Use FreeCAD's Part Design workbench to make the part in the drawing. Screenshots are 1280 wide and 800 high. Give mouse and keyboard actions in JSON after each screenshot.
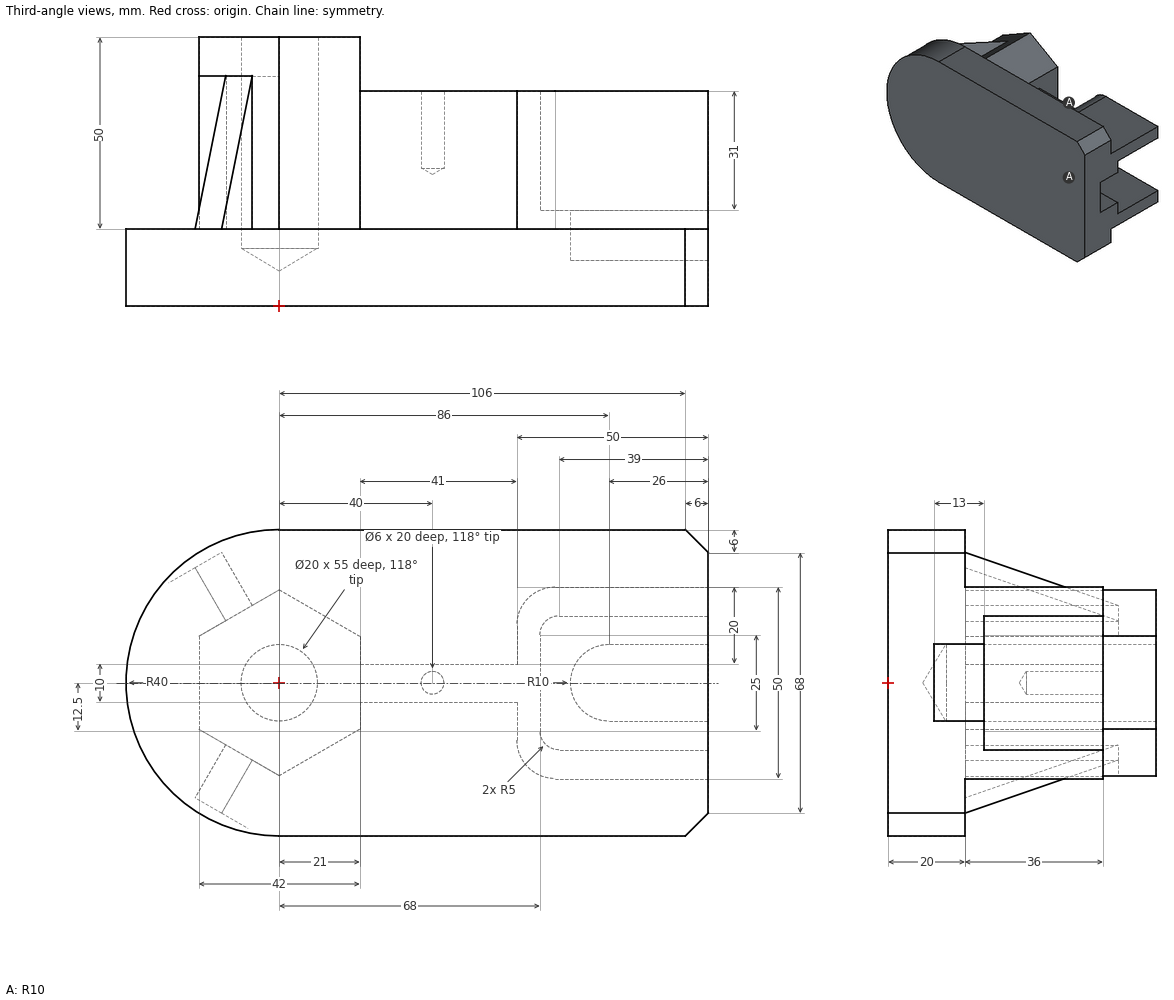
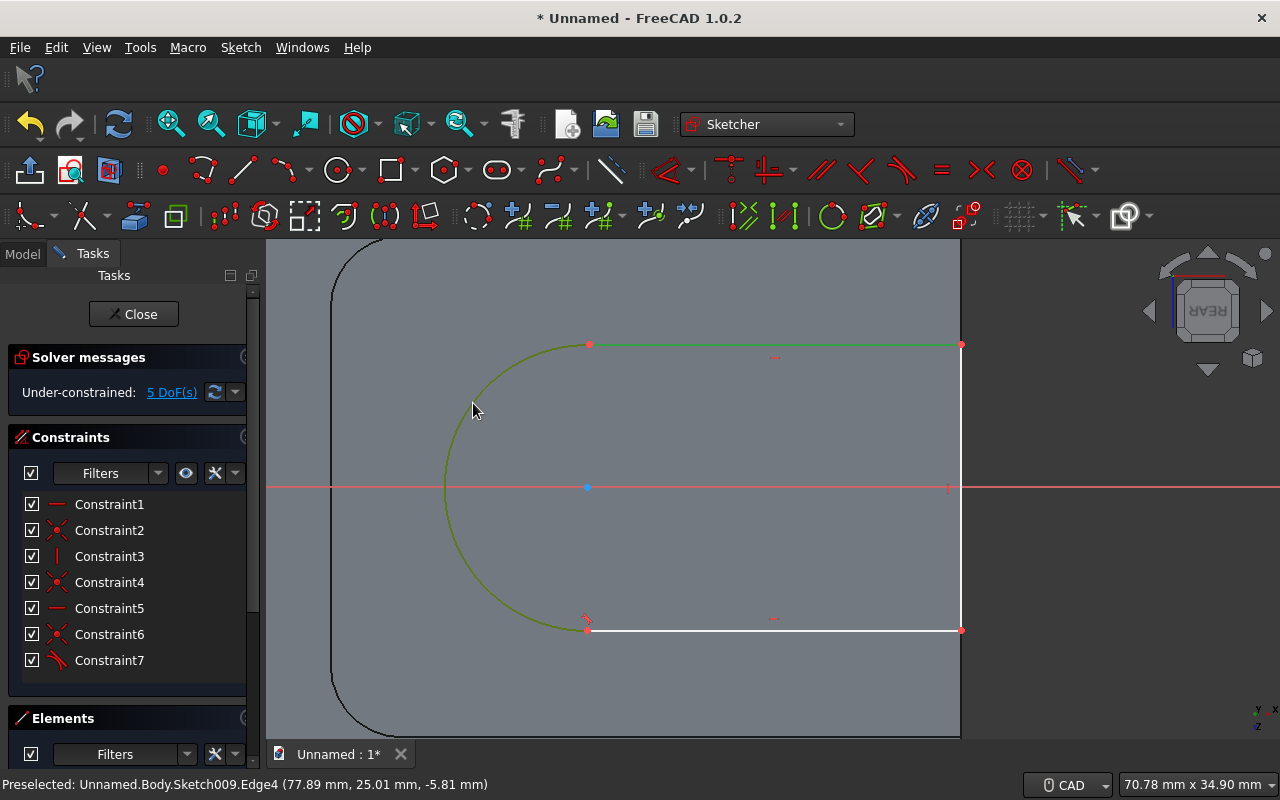
{"action": "left_click", "coordinate": [902, 170]}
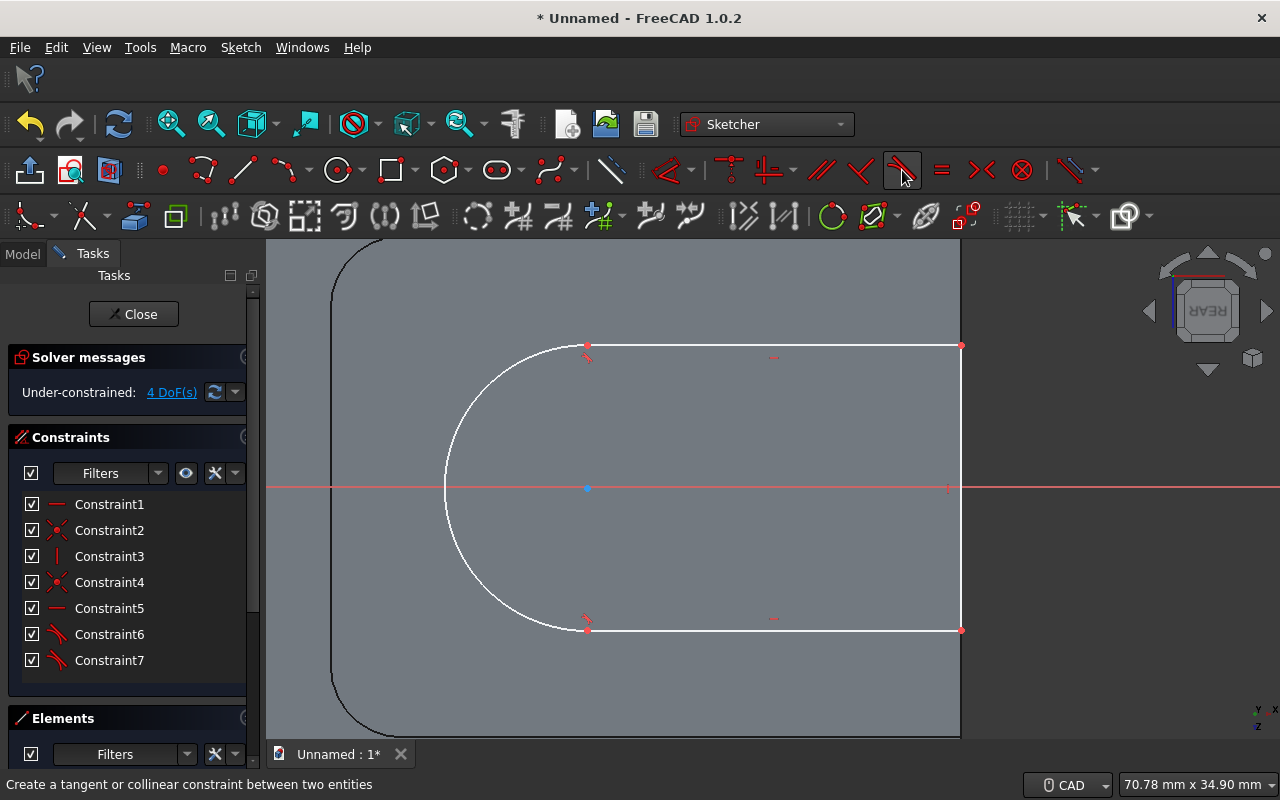
{"action": "left_click", "coordinate": [588, 488]}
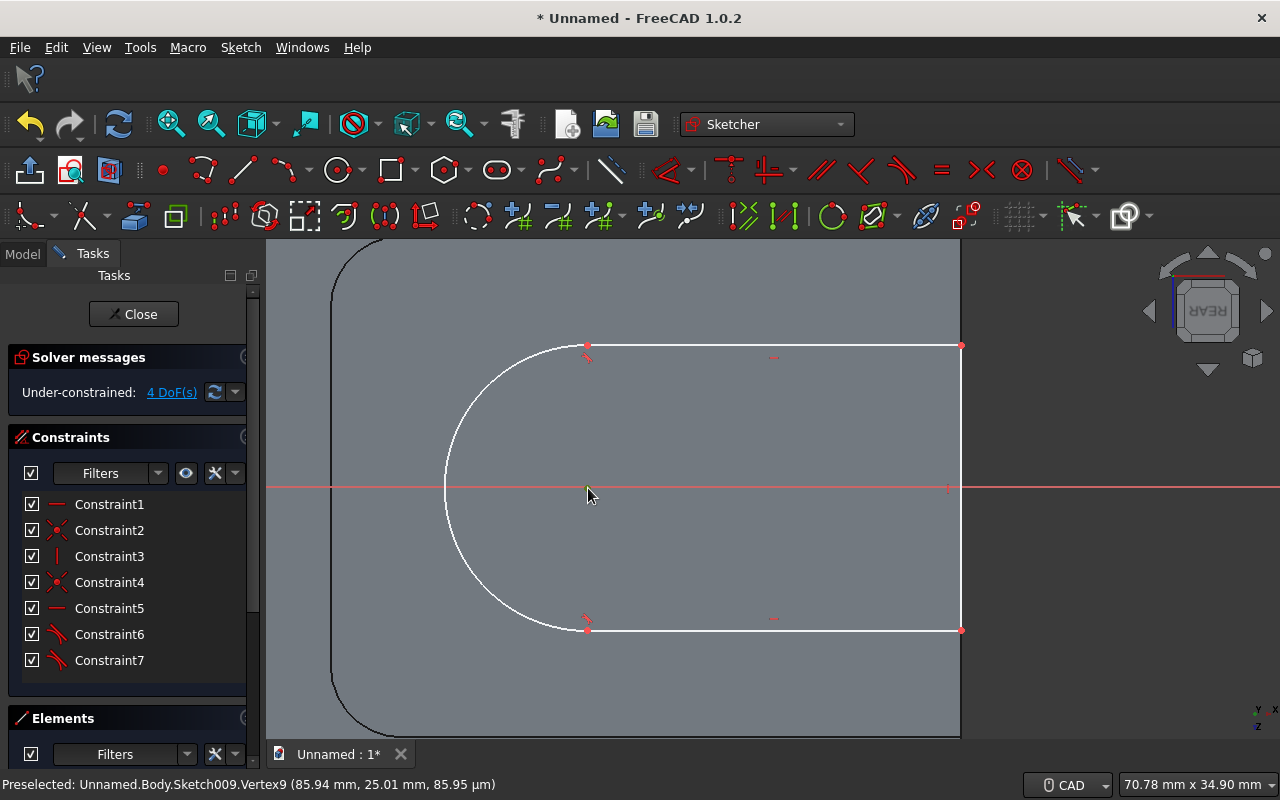
{"action": "left_click", "coordinate": [353, 487]}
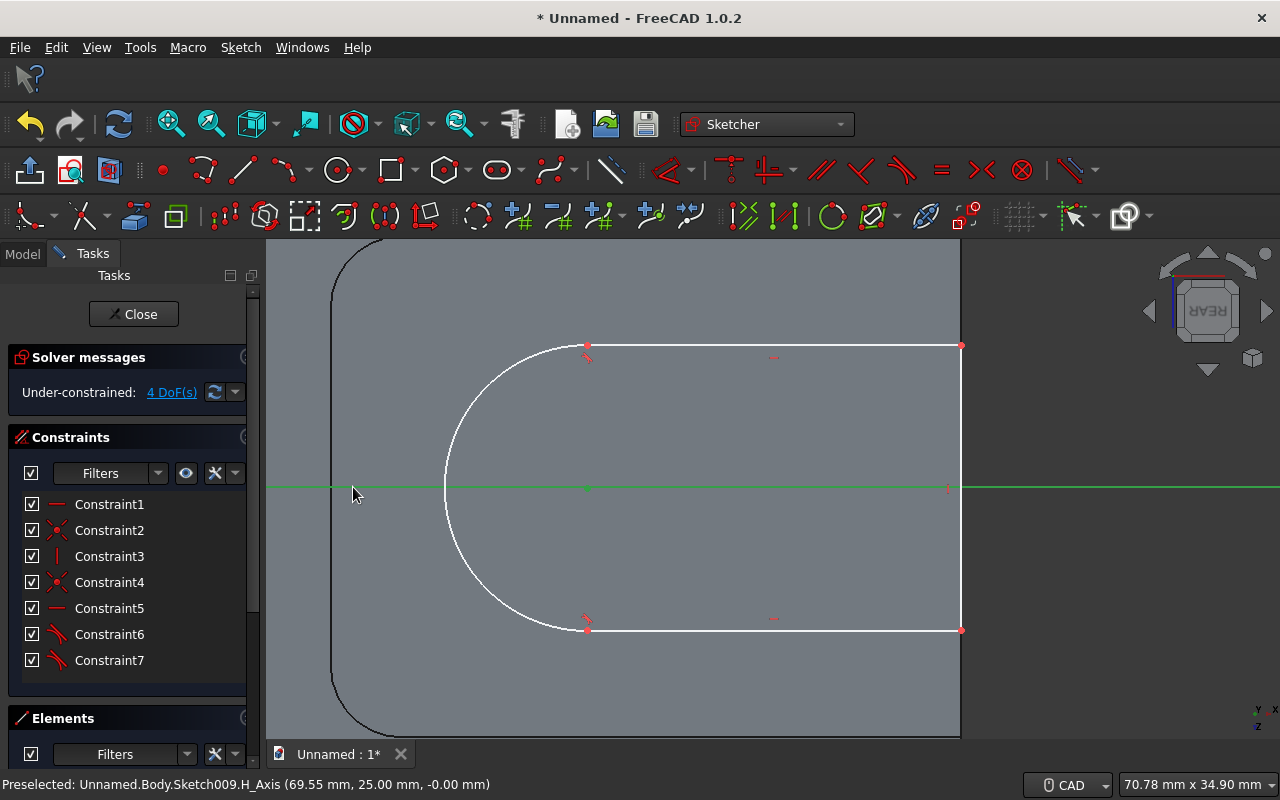
{"action": "left_click", "coordinate": [730, 170]}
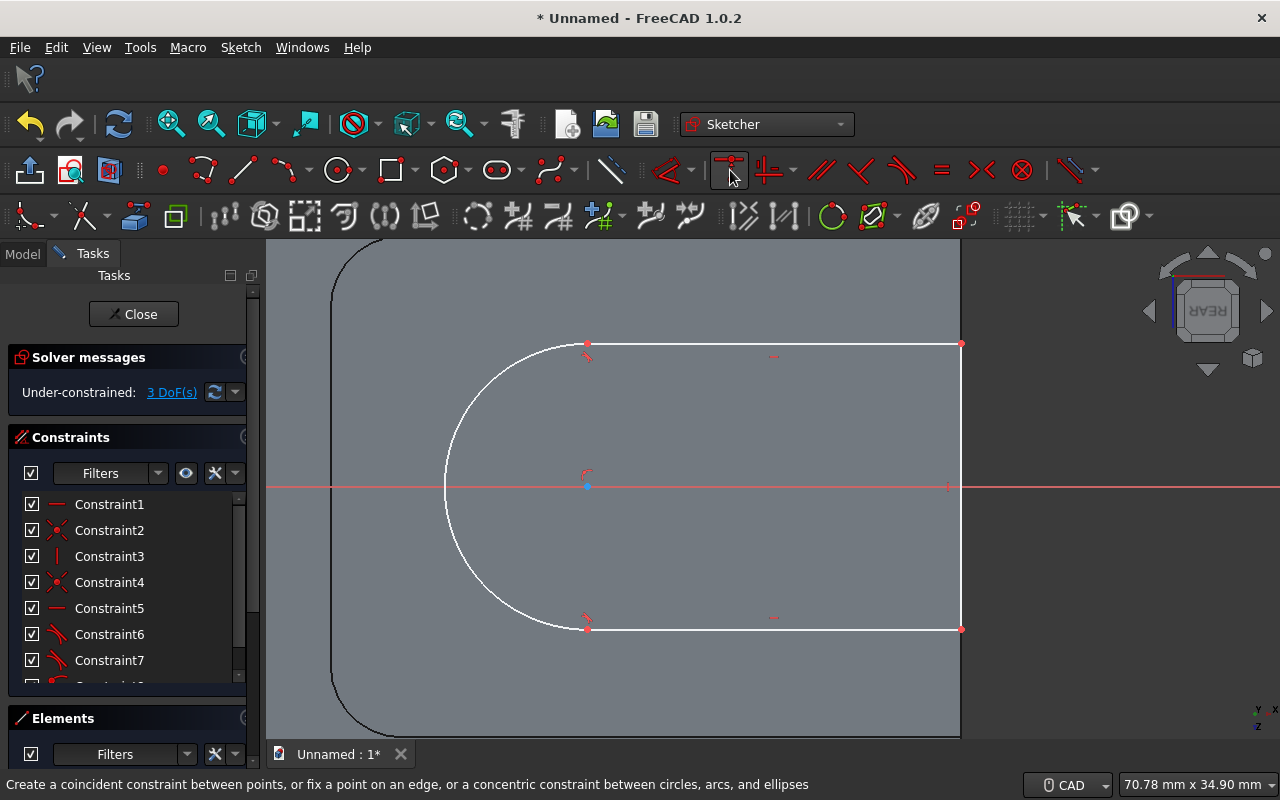
{"action": "left_click", "coordinate": [666, 170]}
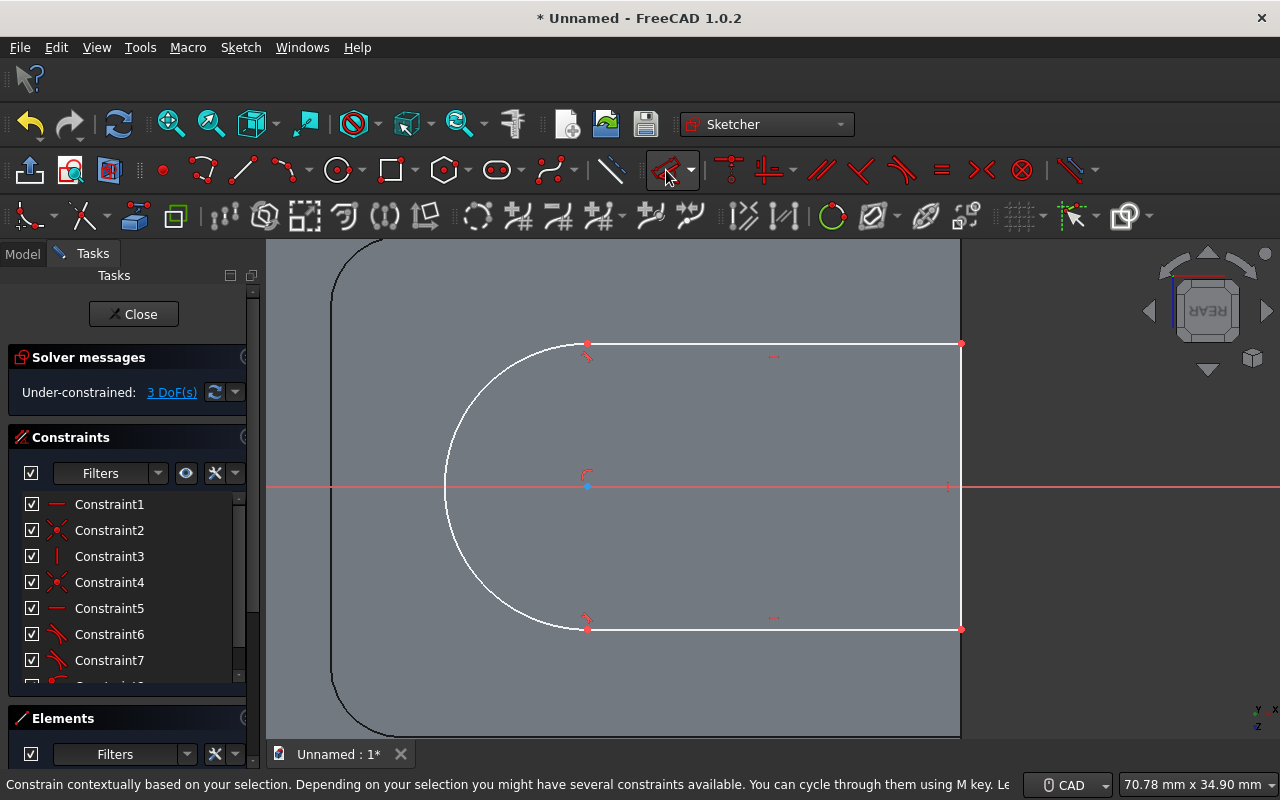
{"action": "left_click", "coordinate": [472, 403]}
{"action": "left_click", "coordinate": [446, 384]}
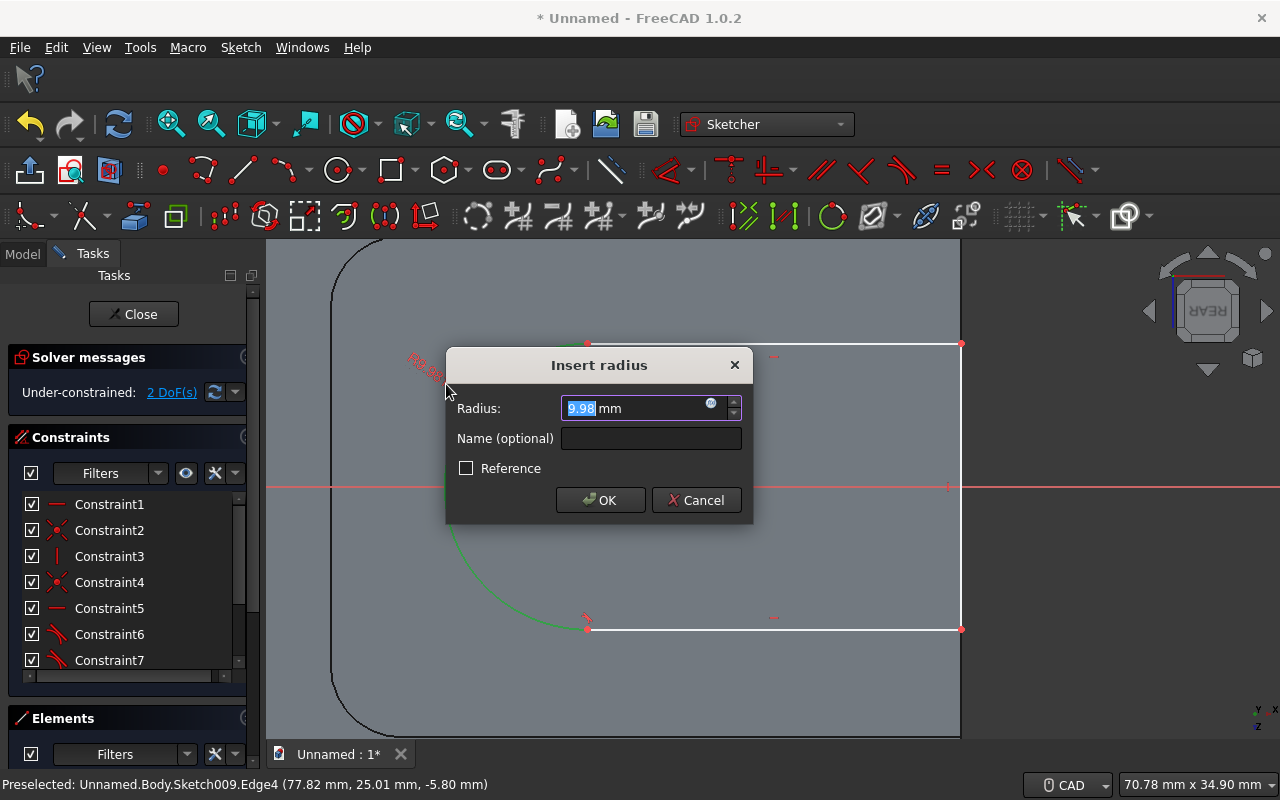
{"action": "type", "text": "10"}
{"action": "key", "text": "Return"}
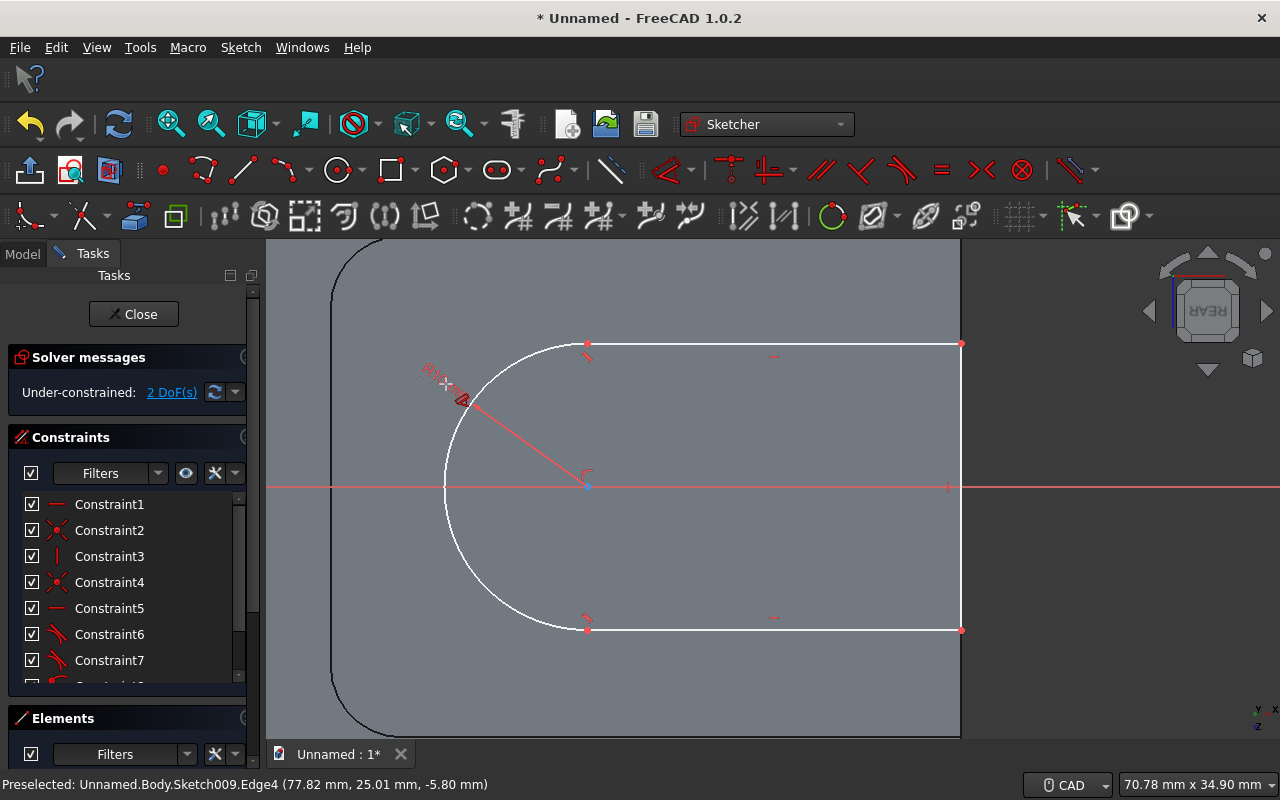
{"action": "left_click", "coordinate": [700, 630]}
{"action": "left_click", "coordinate": [774, 664]}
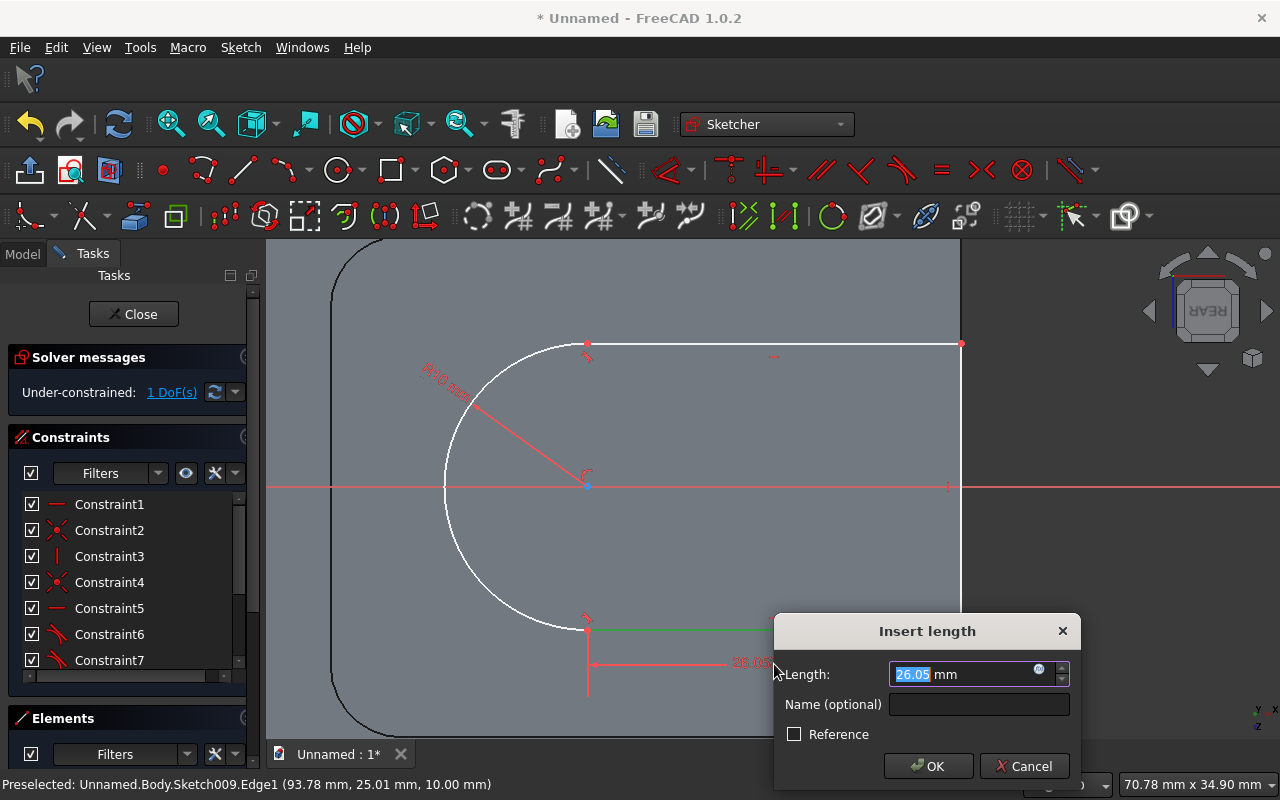
{"action": "type", "text": "26"}
{"action": "key", "text": "Return"}